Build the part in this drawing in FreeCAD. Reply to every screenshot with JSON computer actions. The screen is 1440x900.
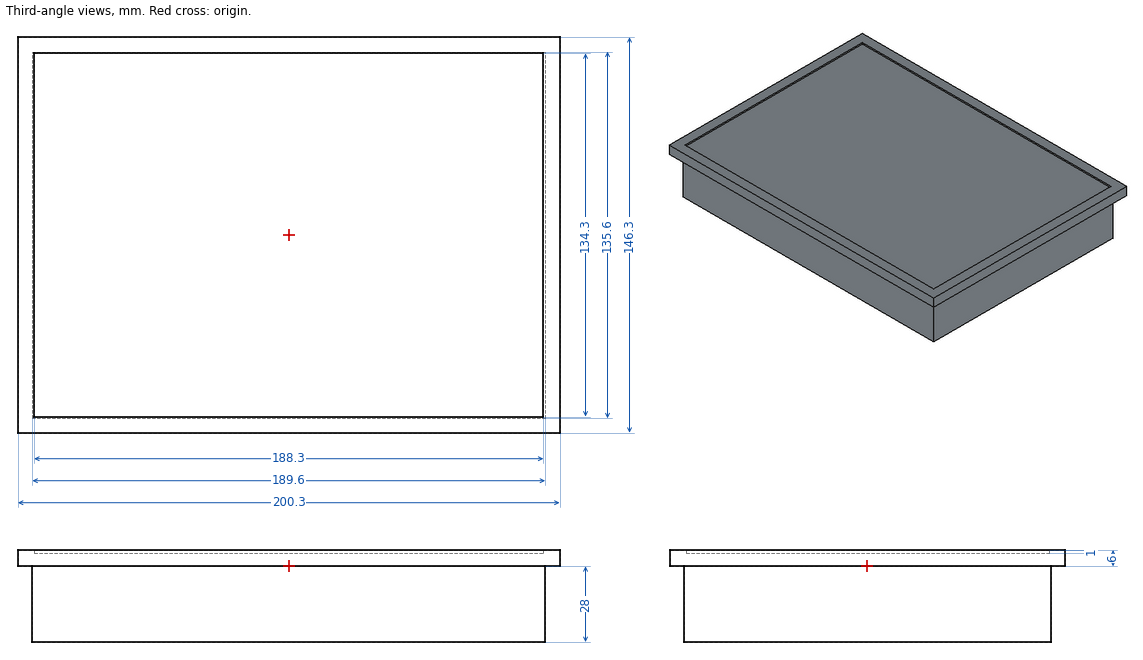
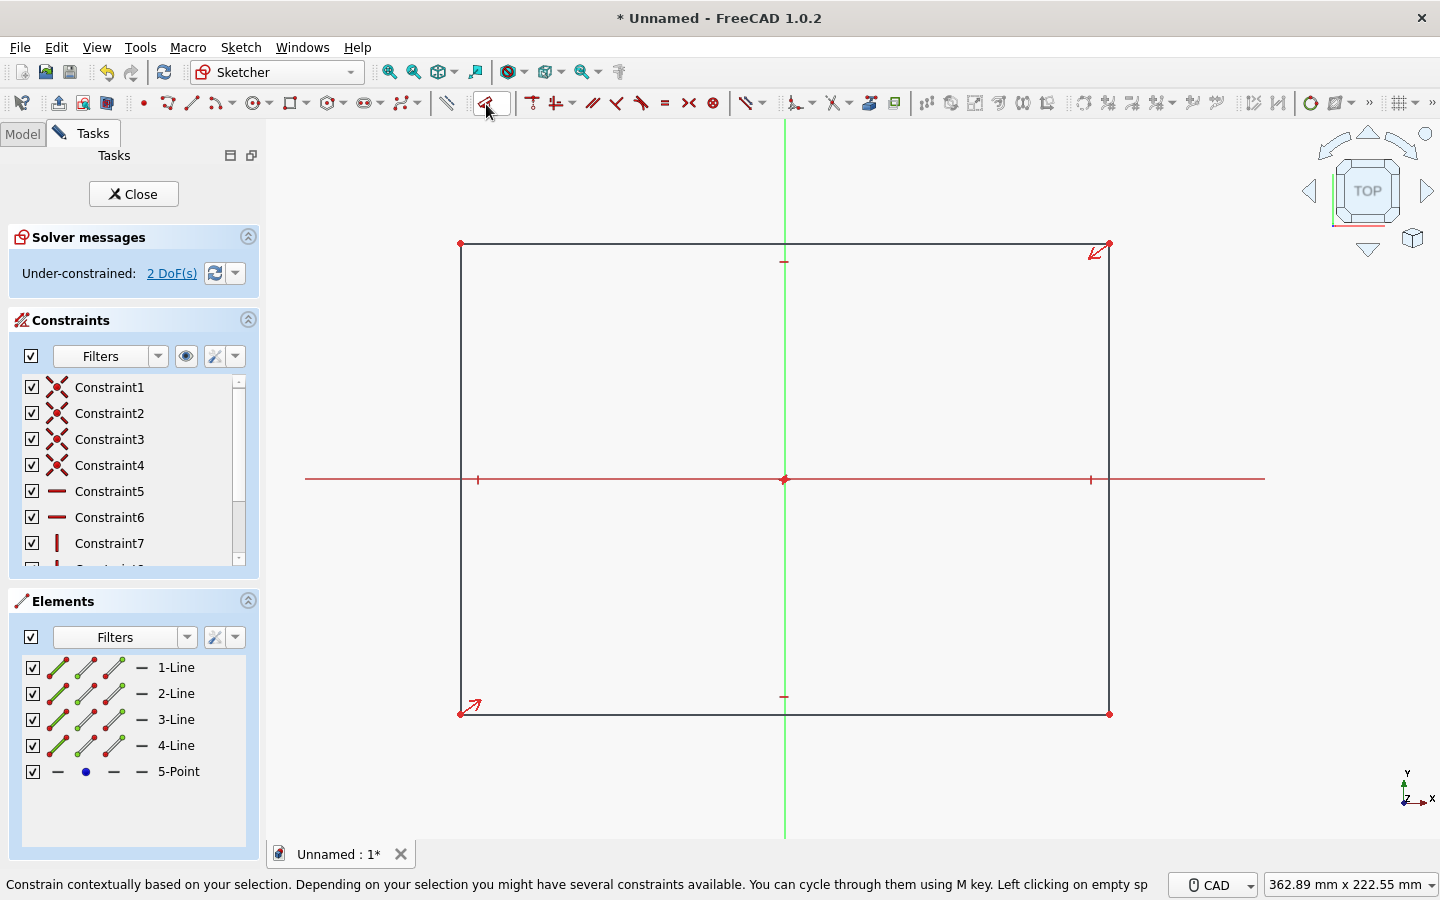
{"action": "left_click", "coordinate": [655, 715]}
{"action": "left_click", "coordinate": [636, 749]}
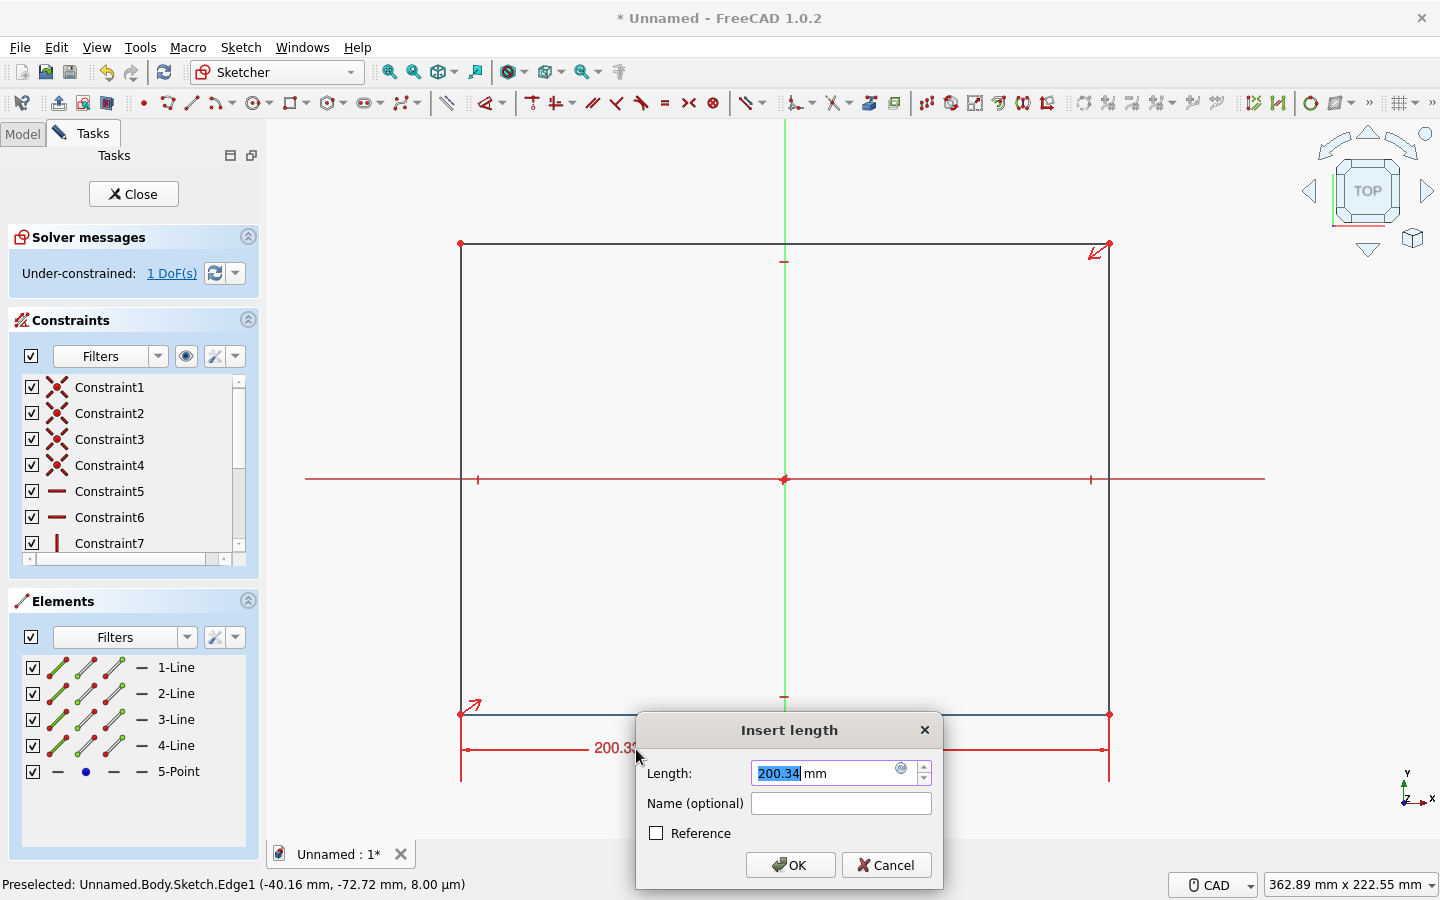
{"action": "type", "text": "200.3"}
{"action": "key", "text": "Return"}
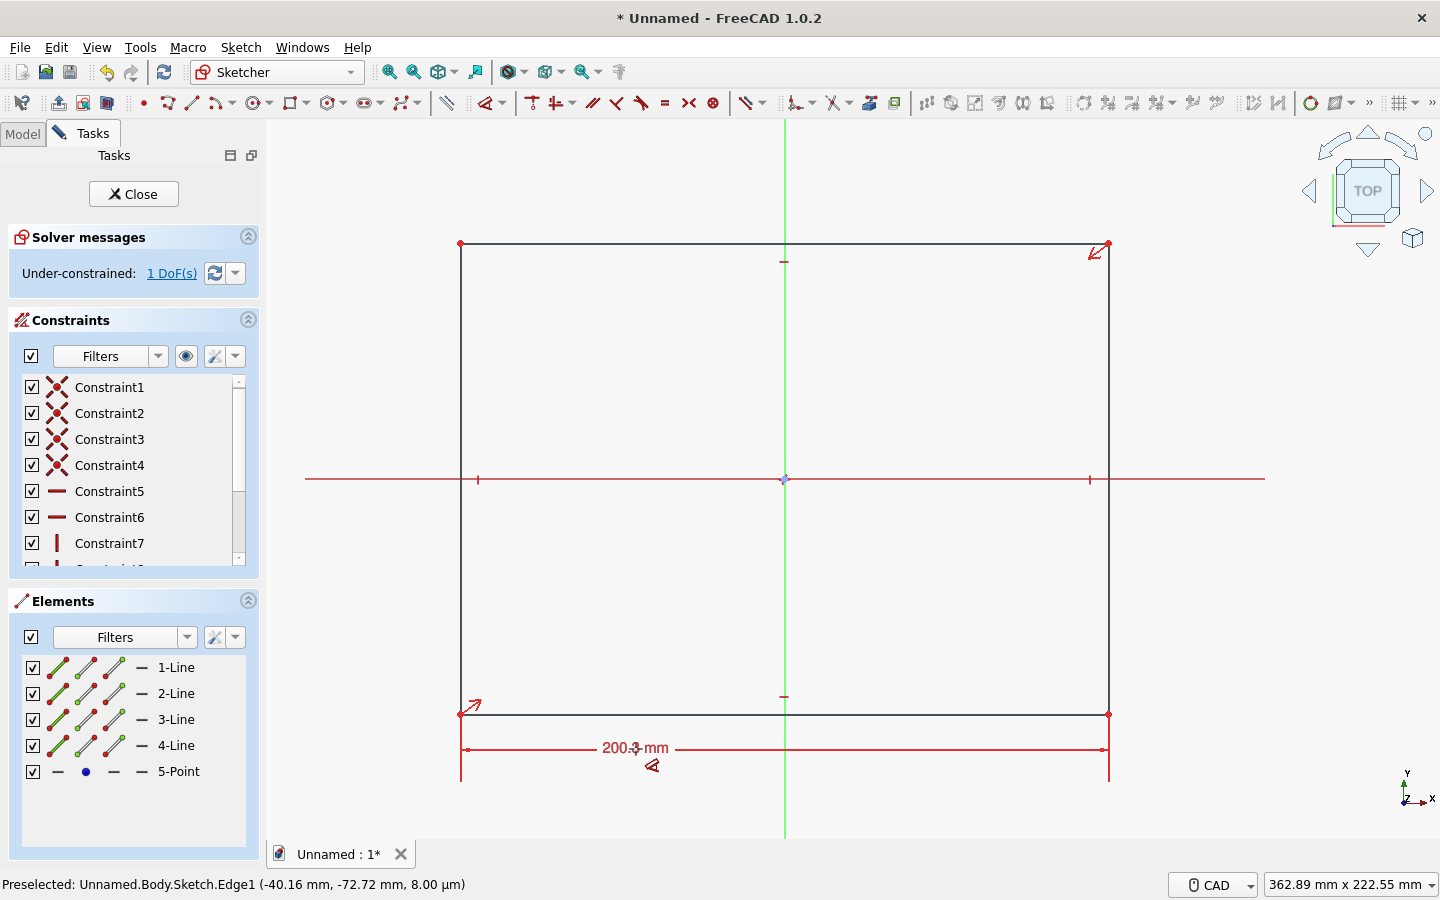
{"action": "left_click", "coordinate": [1109, 573]}
{"action": "left_click", "coordinate": [1143, 371]}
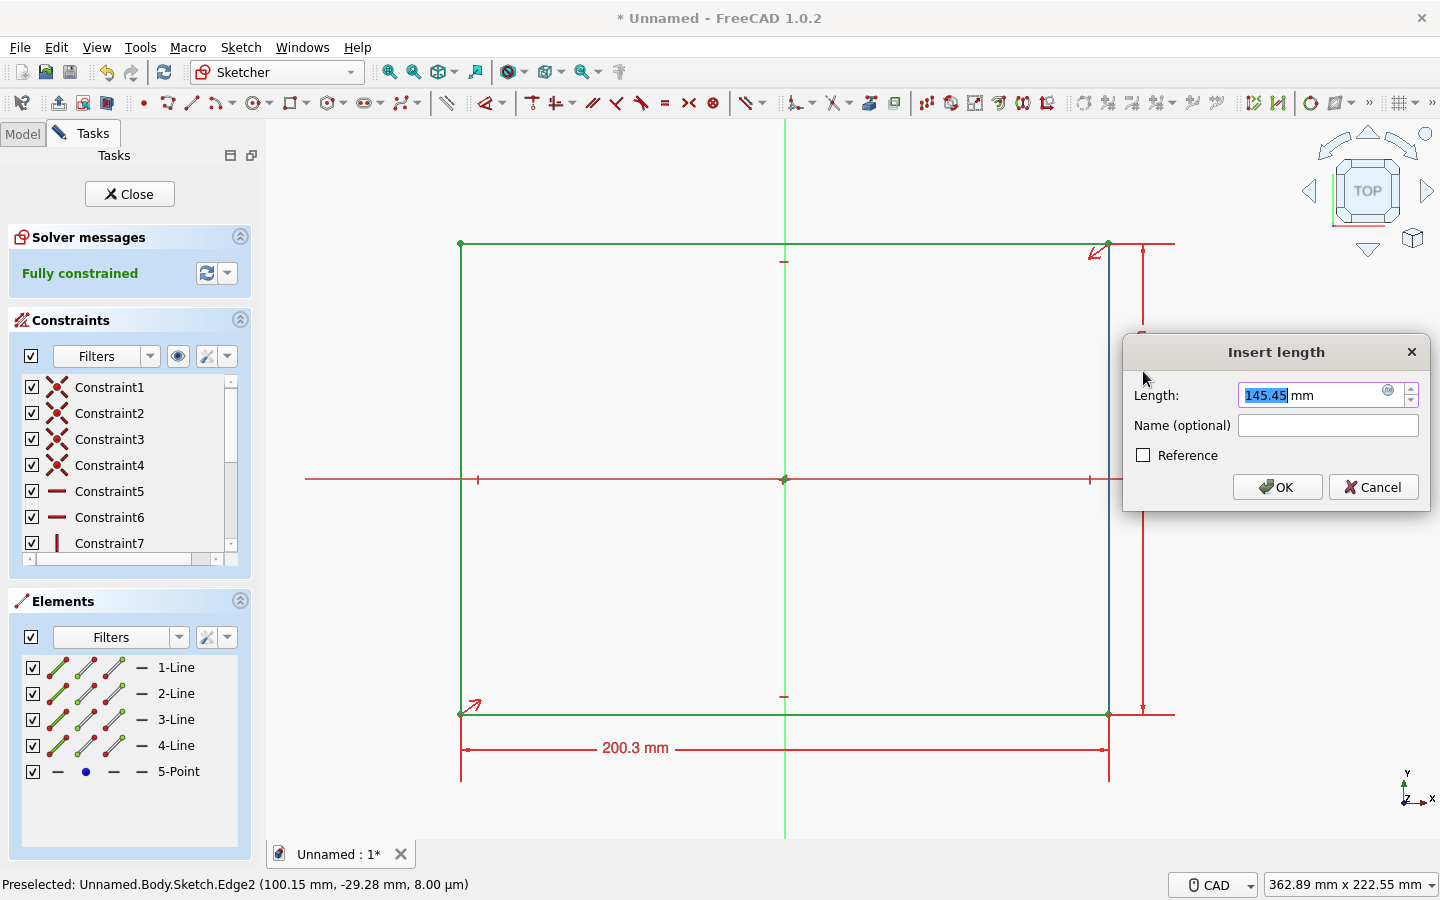
{"action": "type", "text": "146.3"}
{"action": "key", "text": "Return"}
{"action": "key", "text": "Escape"}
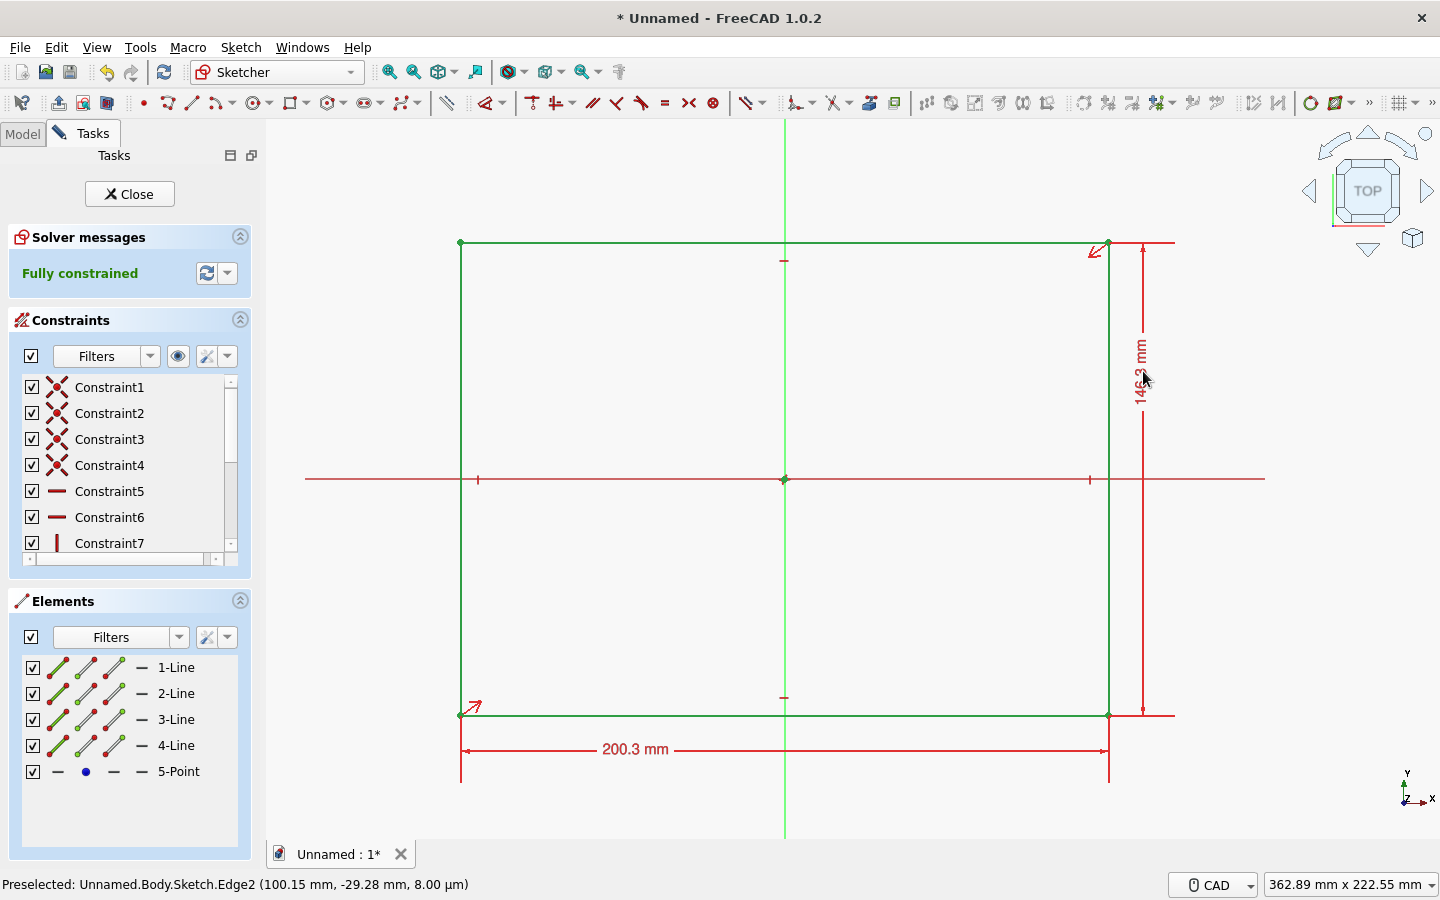
{"action": "left_click", "coordinate": [130, 194]}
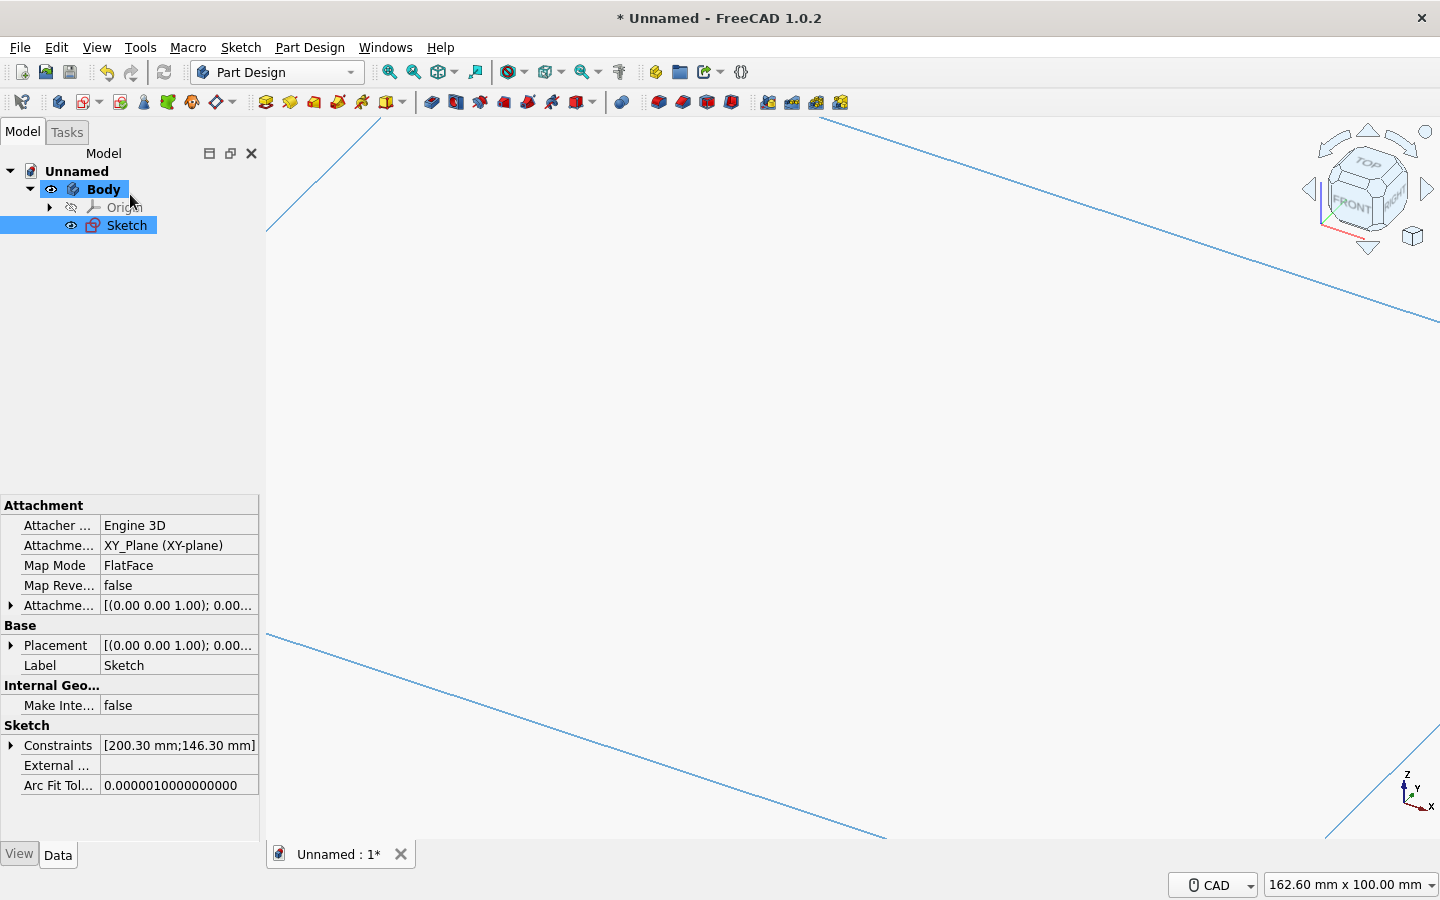
{"action": "left_click", "coordinate": [266, 102]}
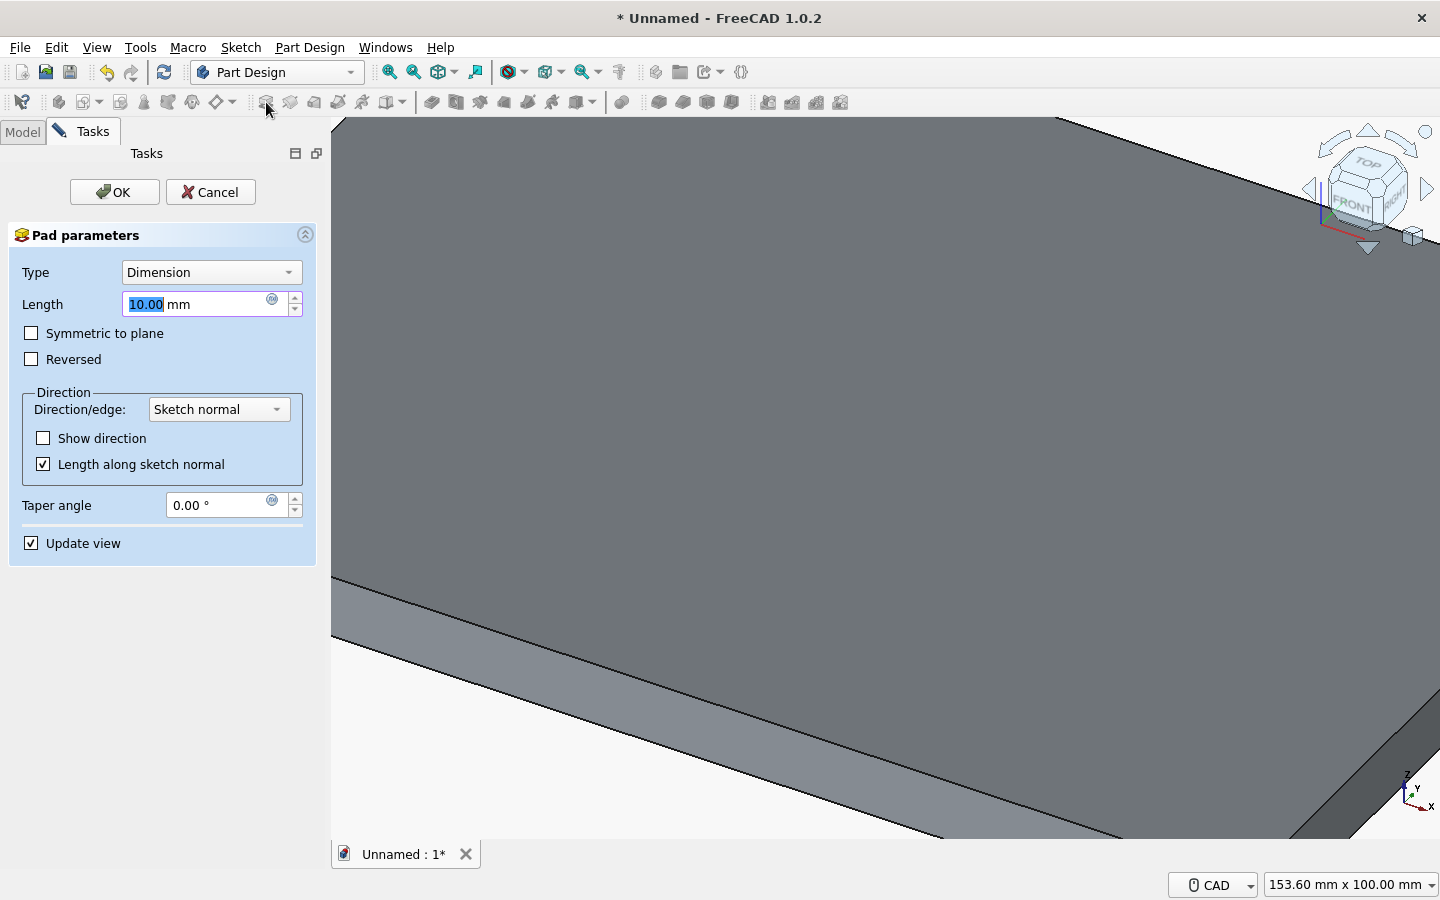
{"action": "type", "text": "6"}
{"action": "key", "text": "Tab"}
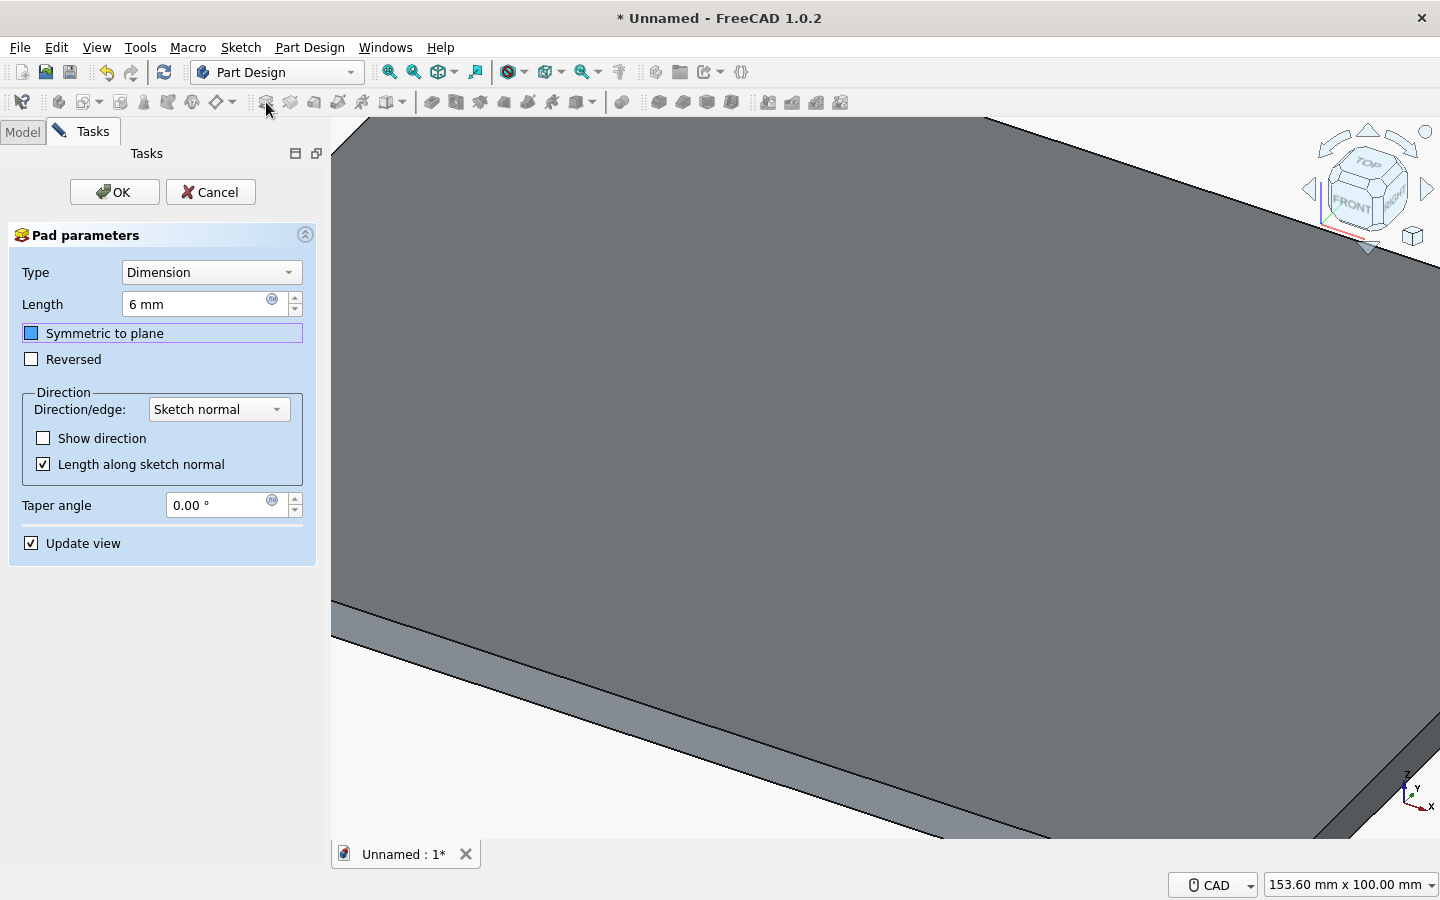
{"action": "left_click", "coordinate": [115, 192]}